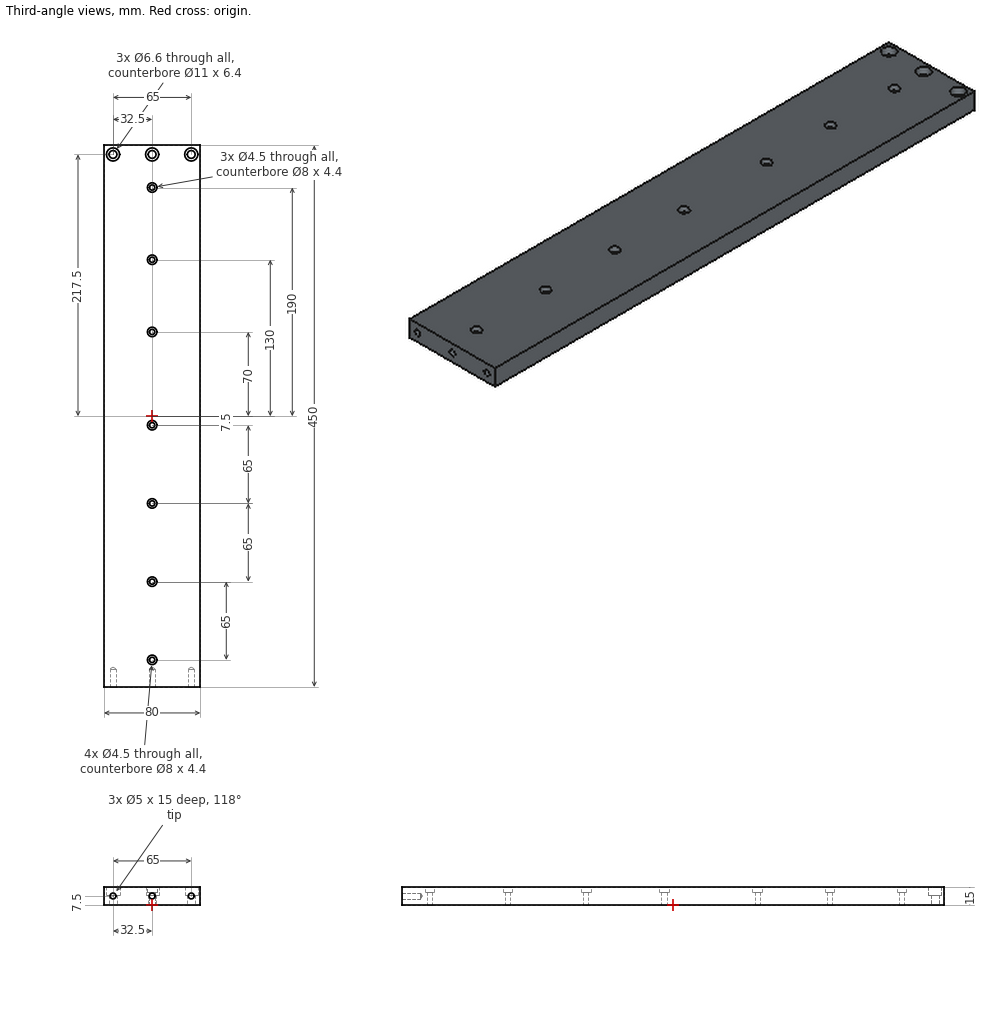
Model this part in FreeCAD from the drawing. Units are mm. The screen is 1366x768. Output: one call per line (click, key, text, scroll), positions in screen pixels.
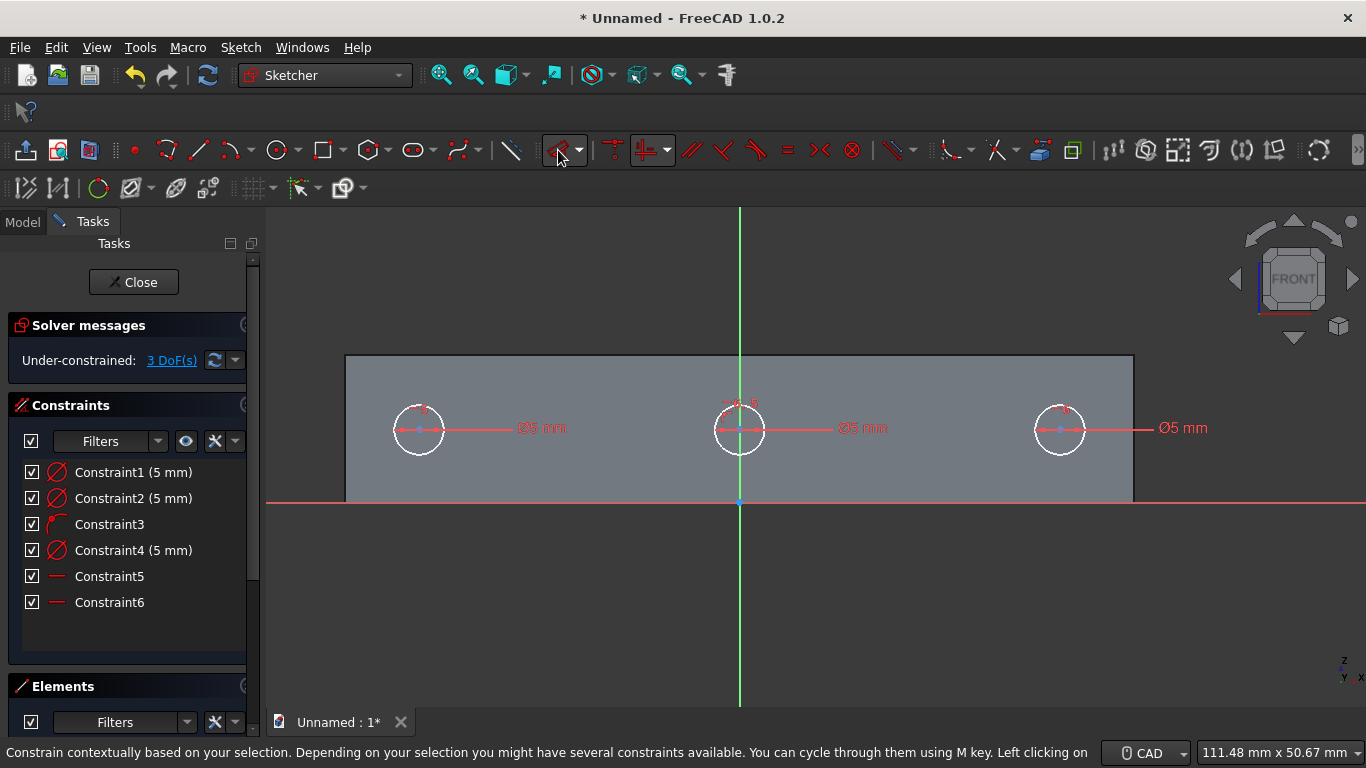
click(419, 430)
click(385, 466)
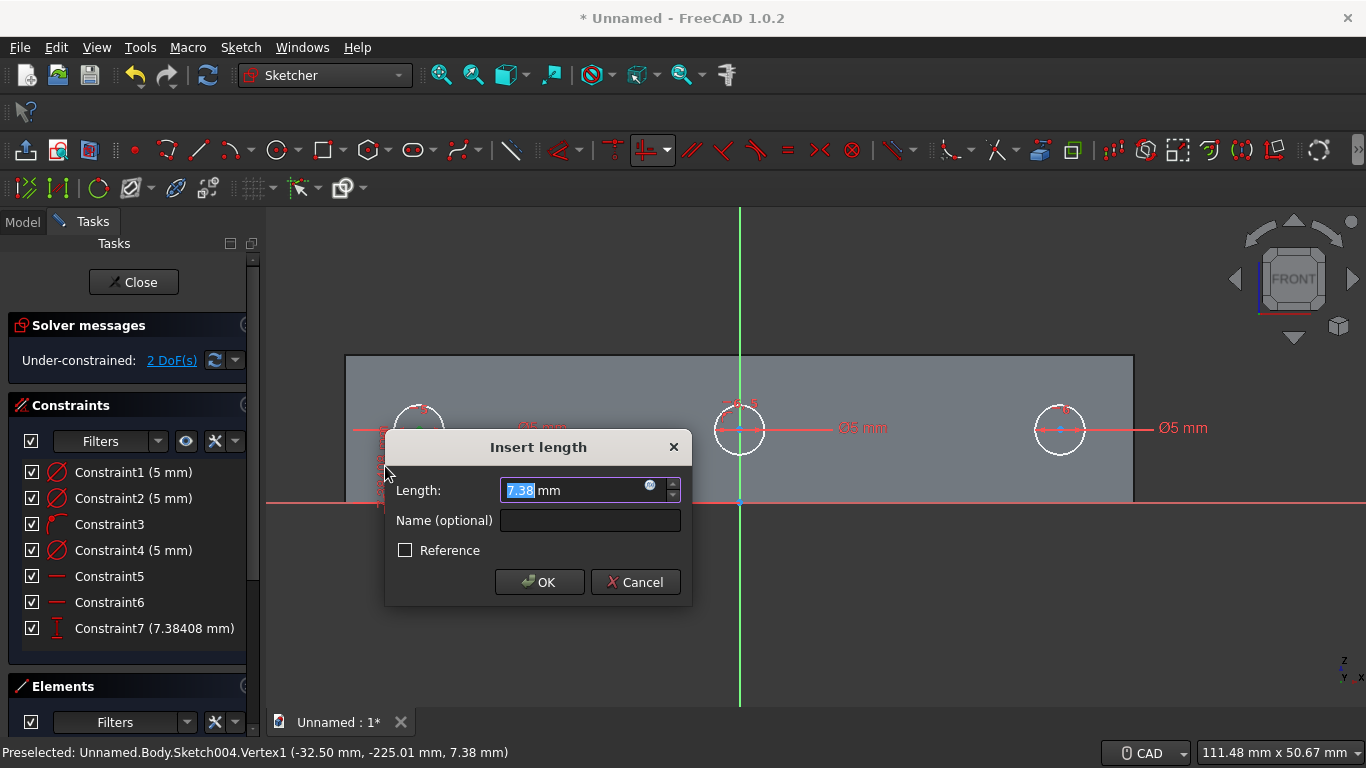
text(7.5)
key(Return)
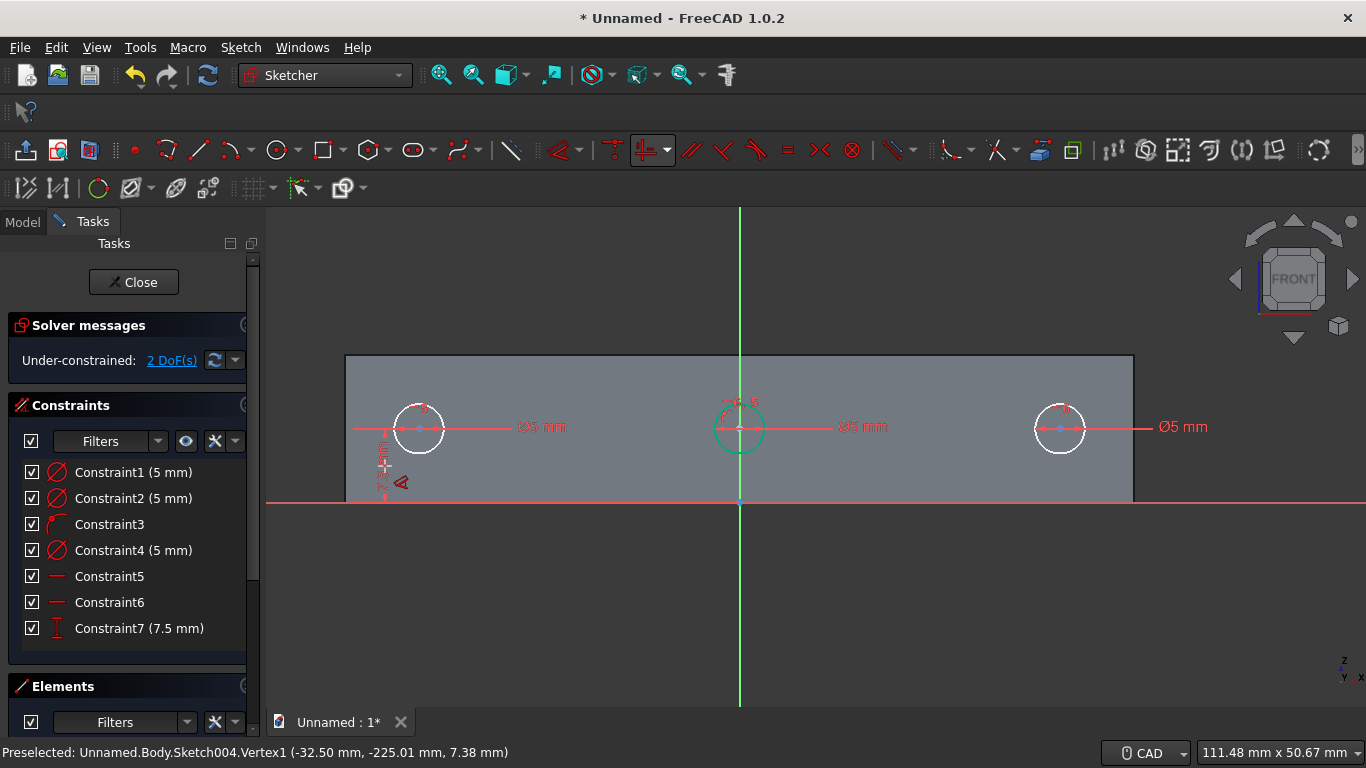
click(419, 429)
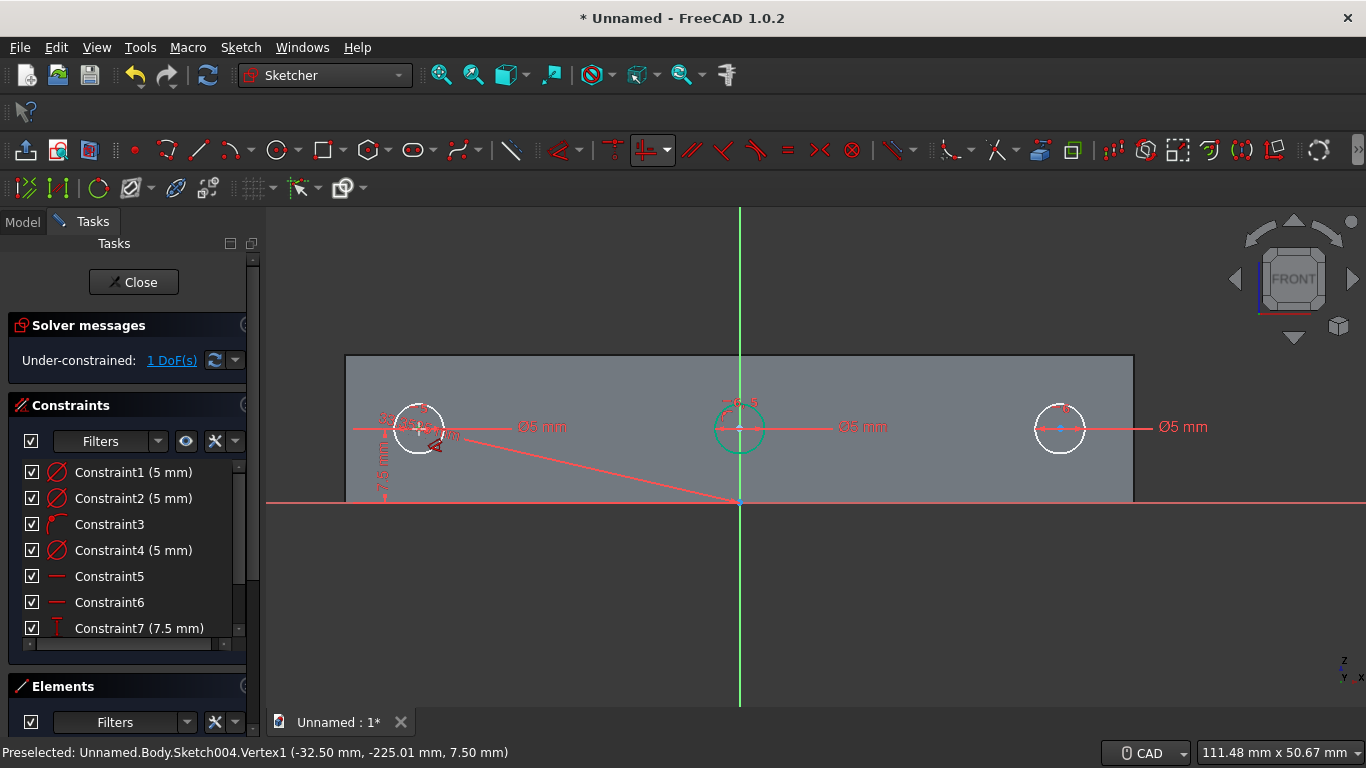
click(1060, 429)
click(592, 395)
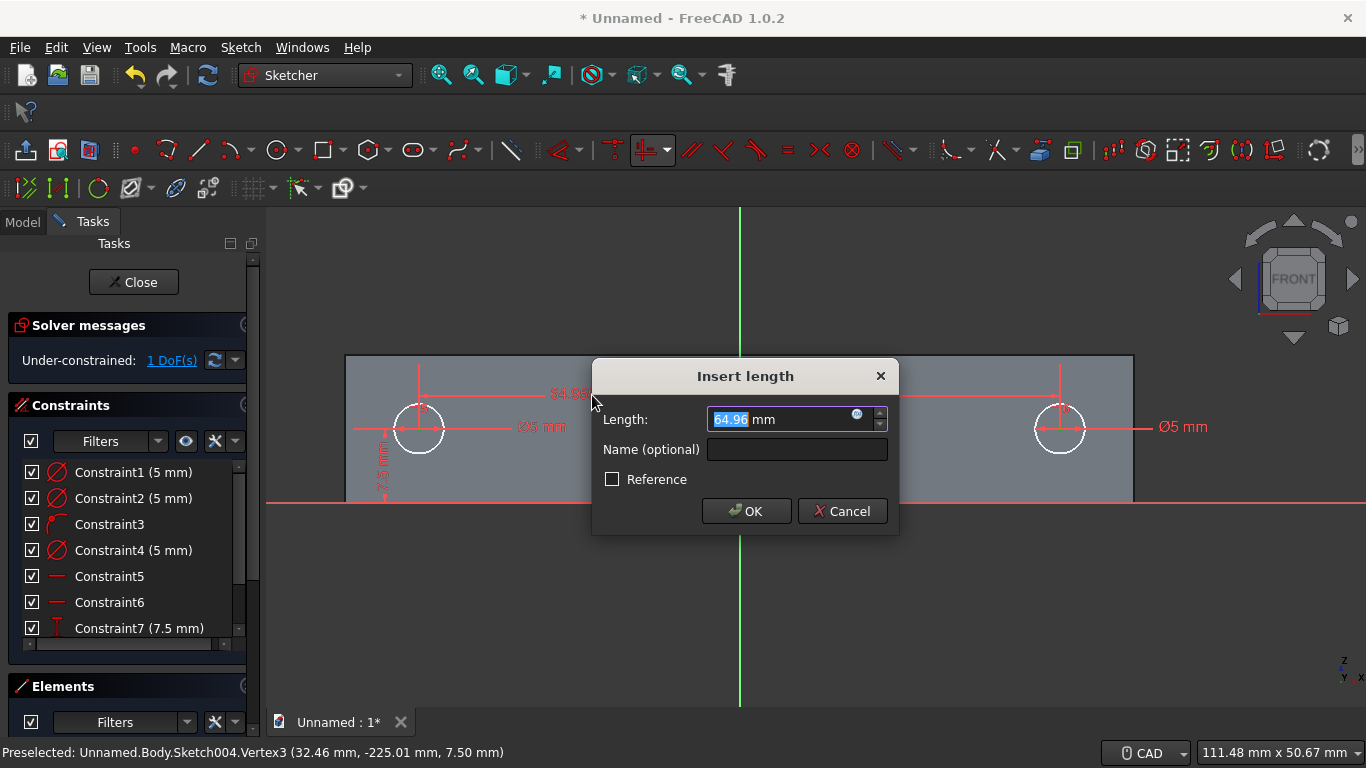
text(65)
key(Return)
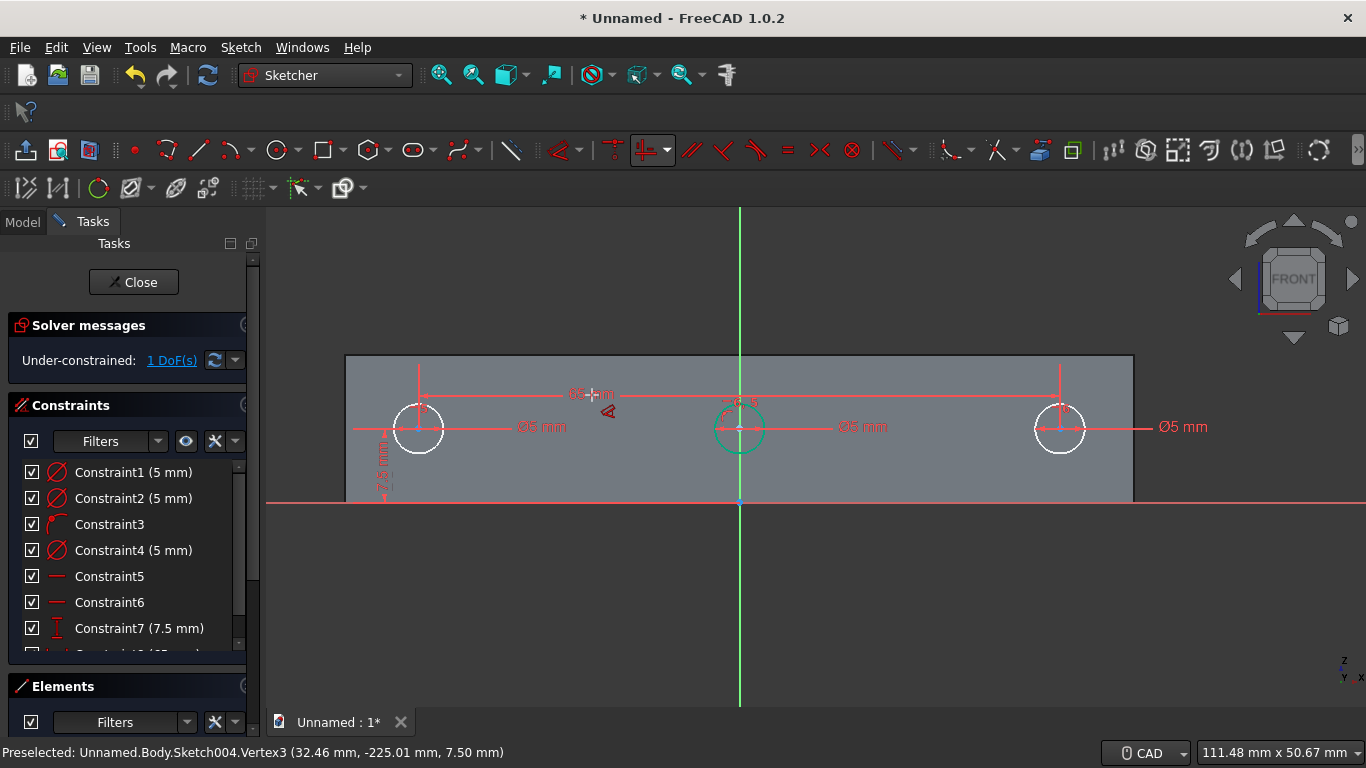
click(419, 429)
click(579, 537)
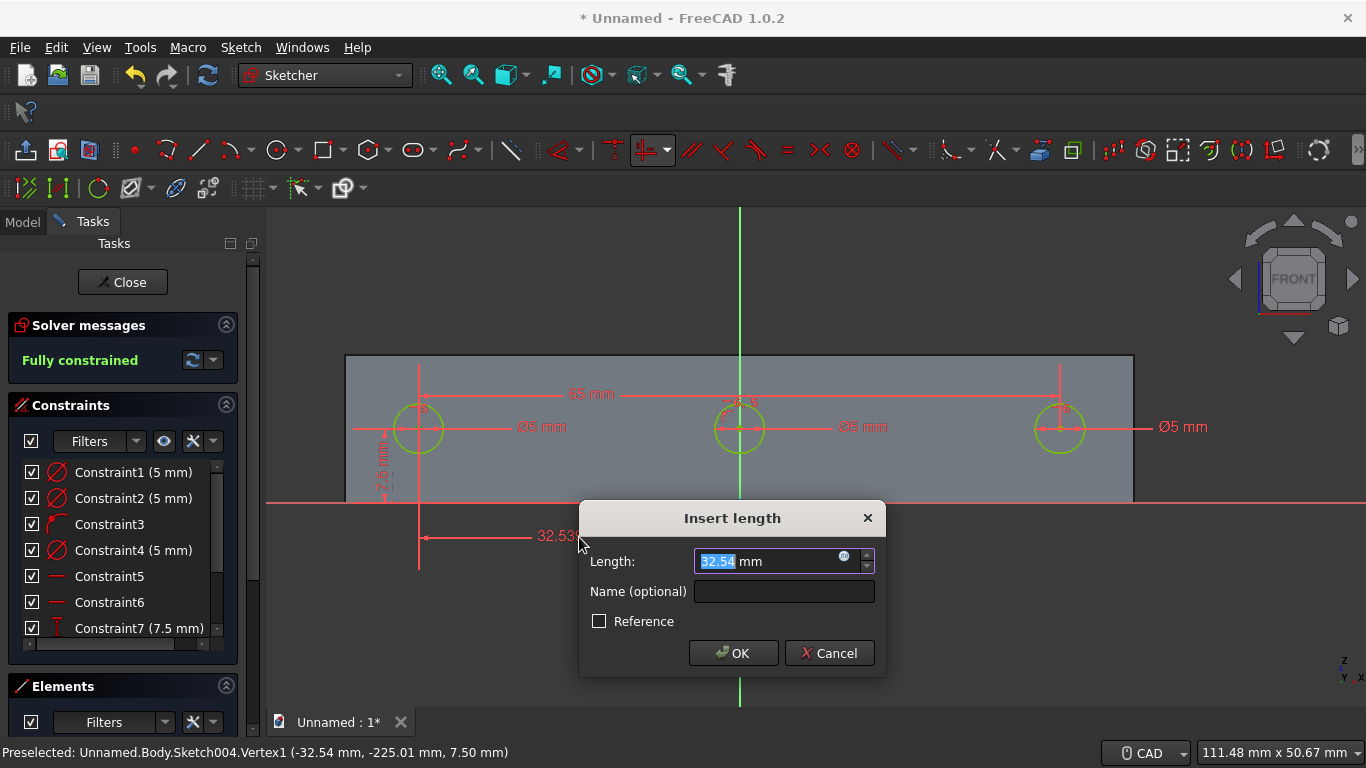
text(32.5)
key(Return)
key(Escape)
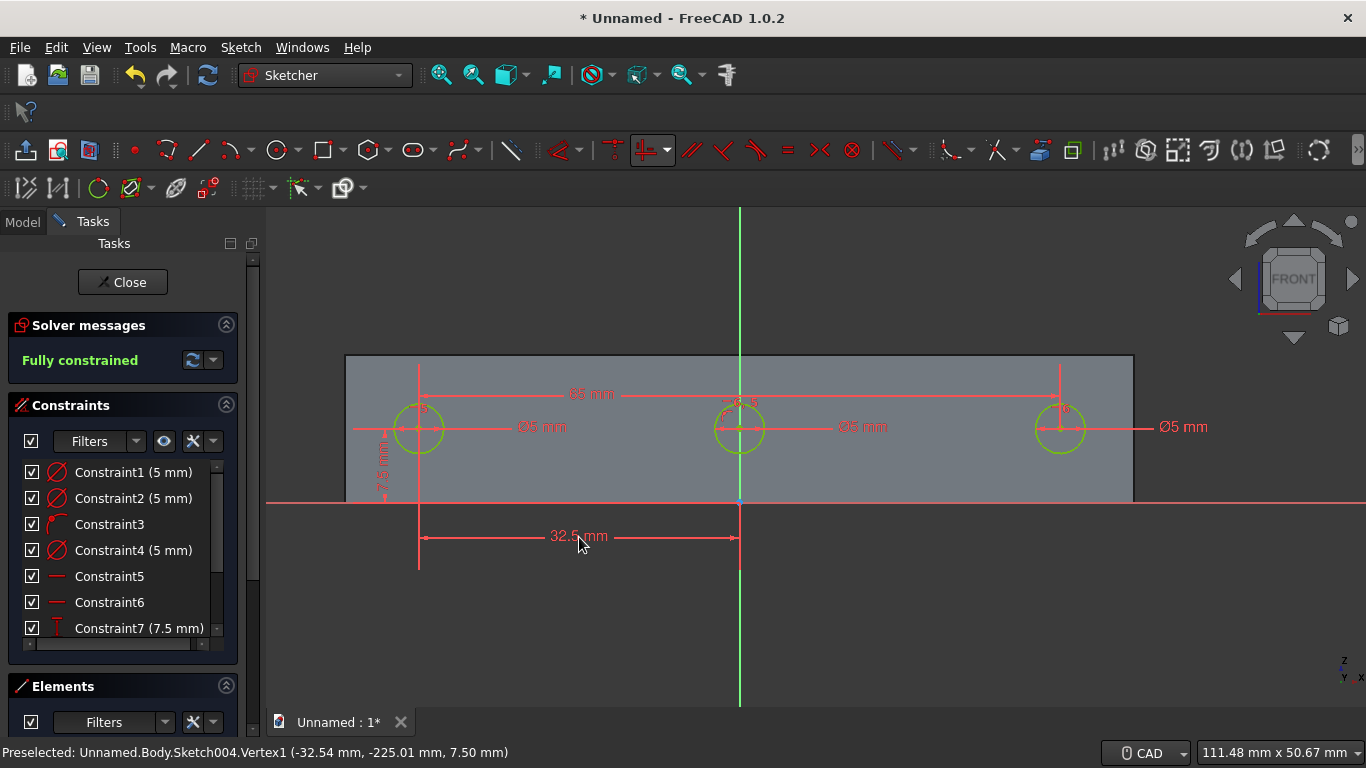
click(123, 282)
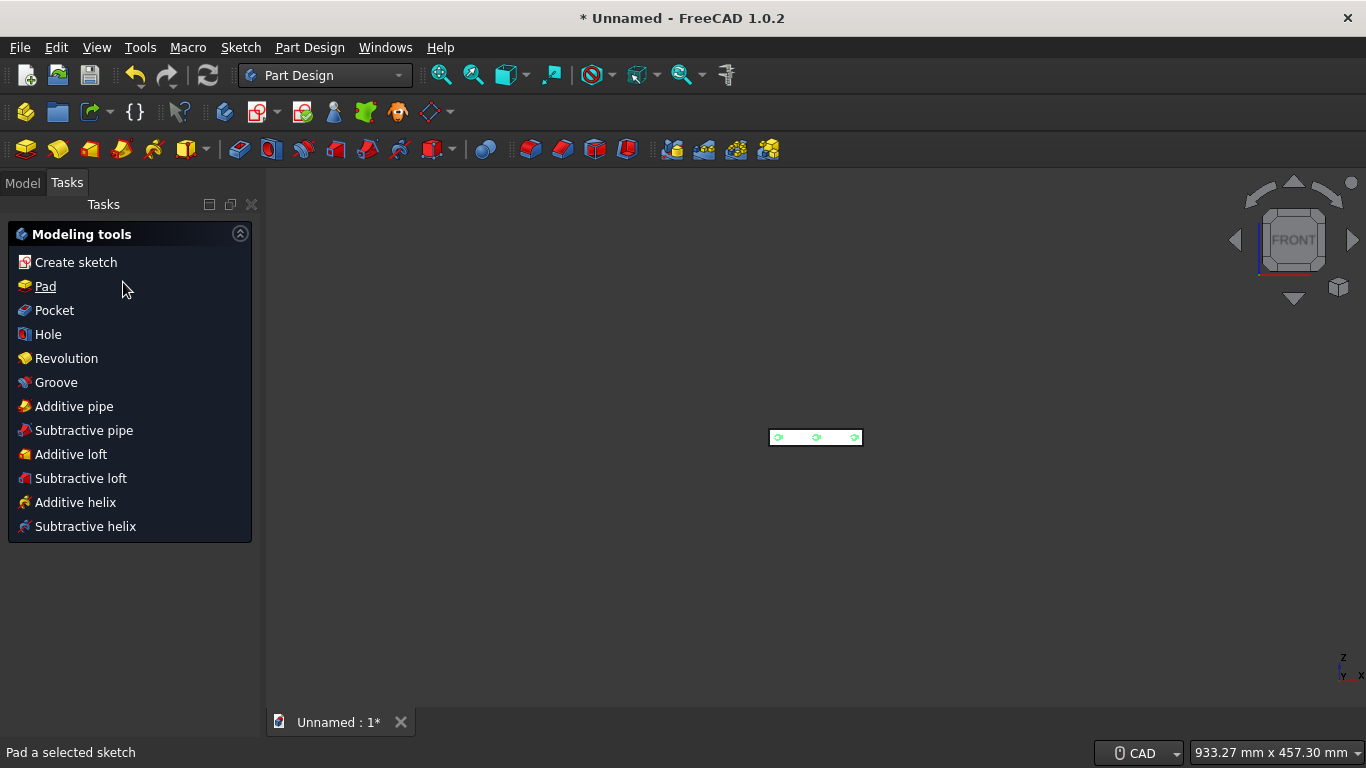
click(272, 150)